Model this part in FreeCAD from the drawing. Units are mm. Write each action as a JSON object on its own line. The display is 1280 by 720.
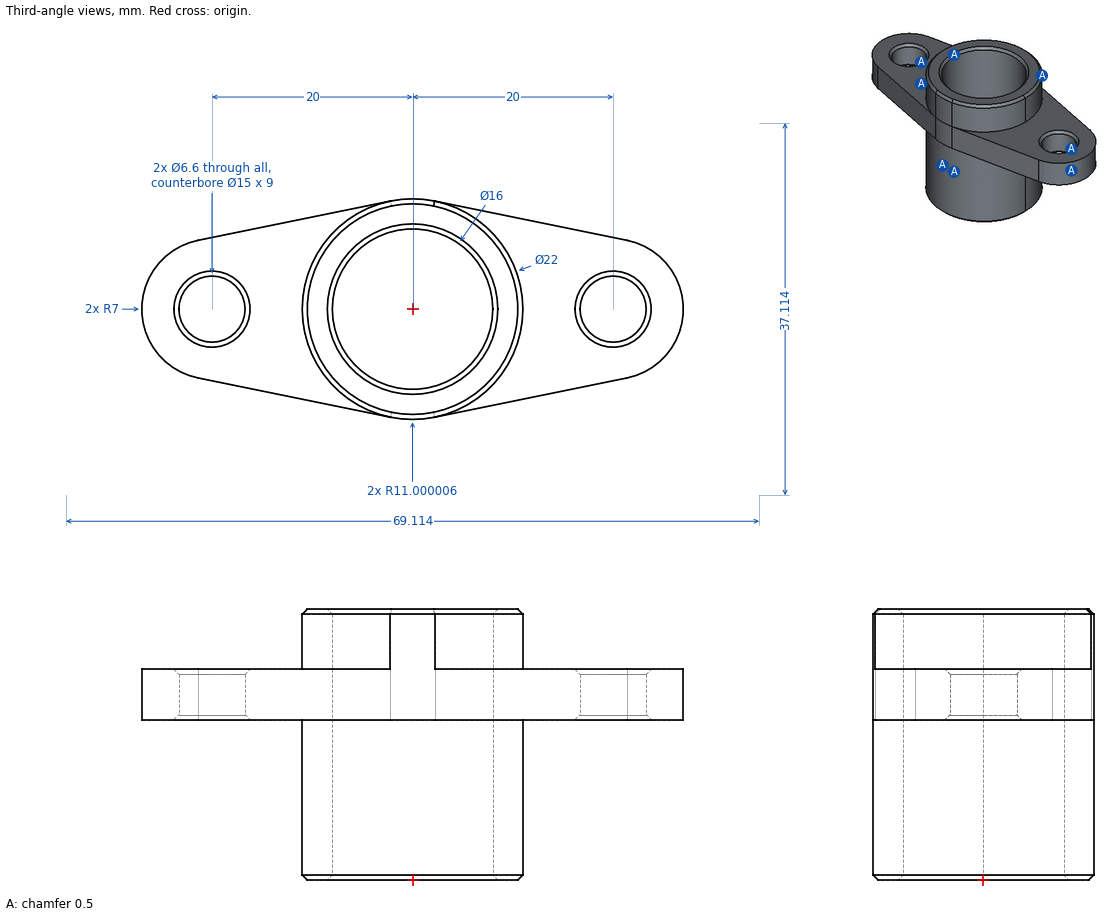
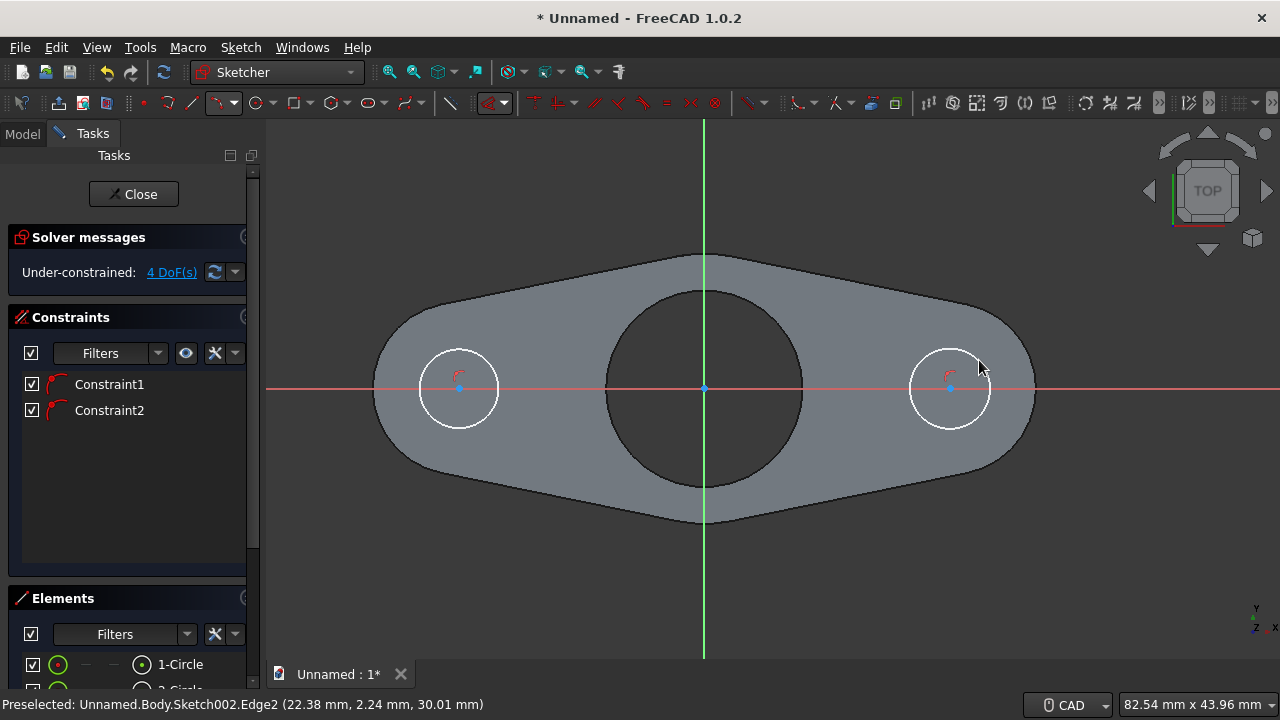
{"action": "left_click", "coordinate": [487, 361]}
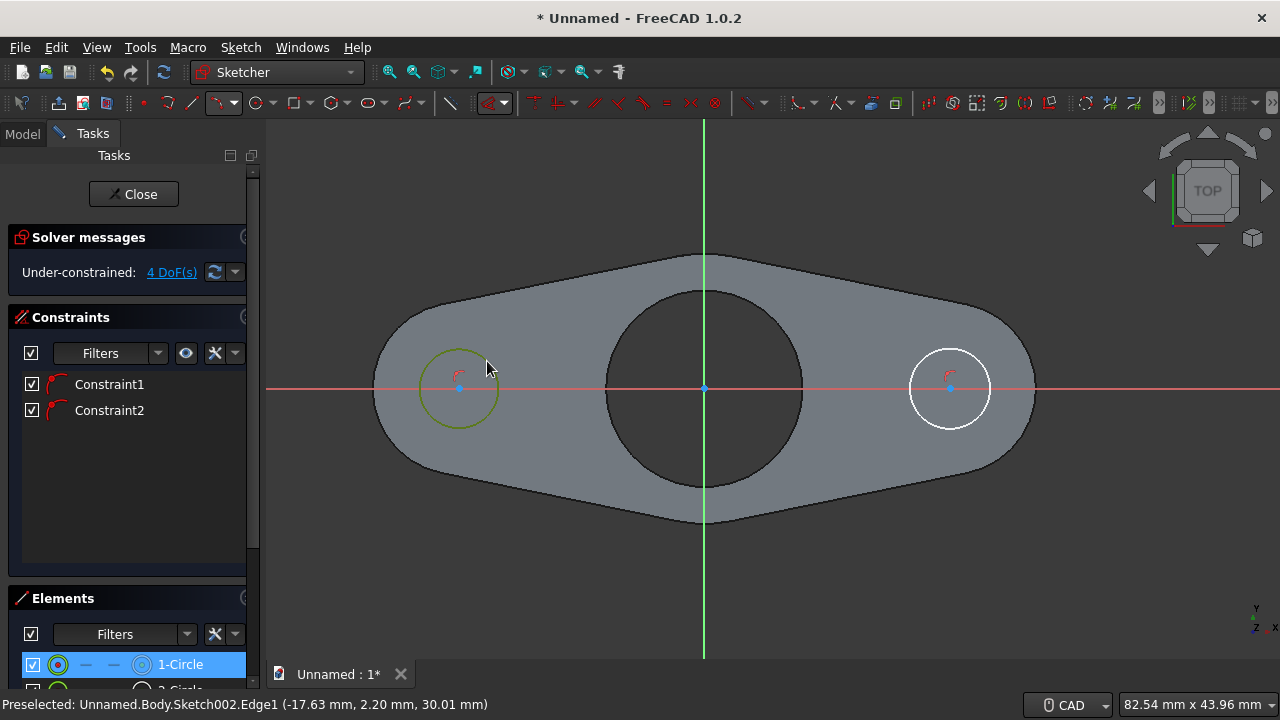
{"action": "left_click", "coordinate": [978, 360]}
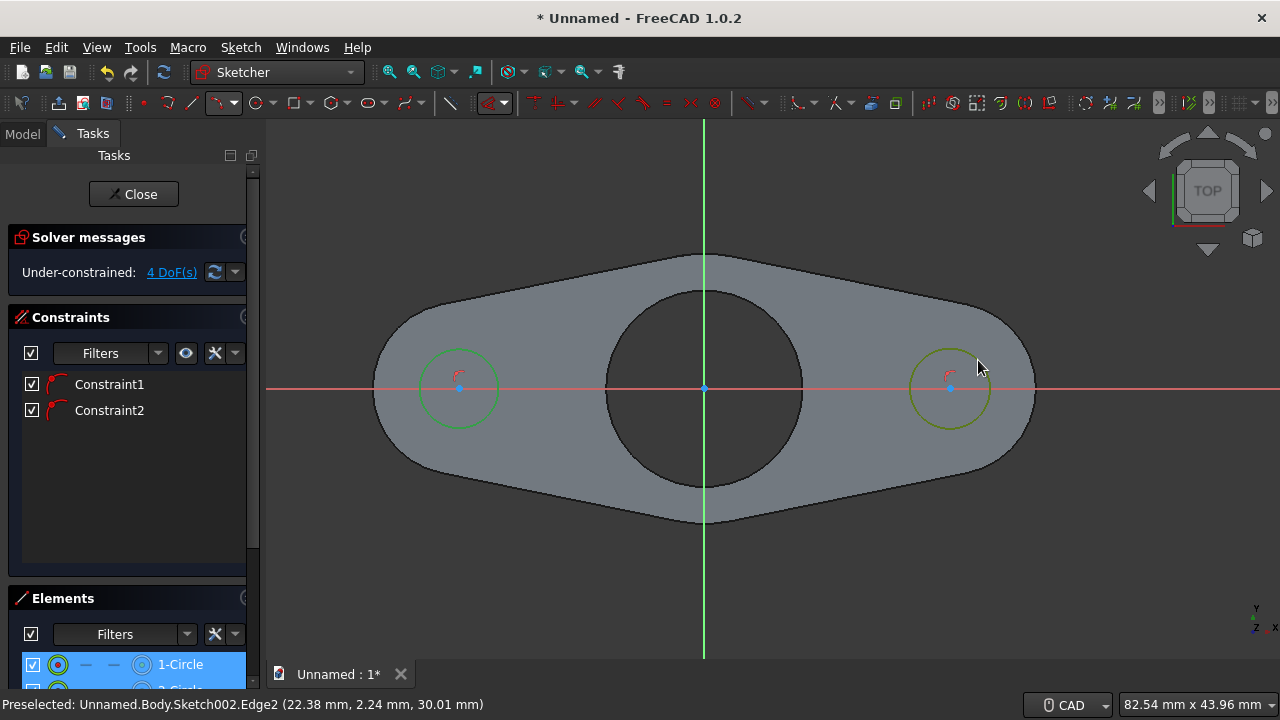
{"action": "left_click", "coordinate": [668, 104]}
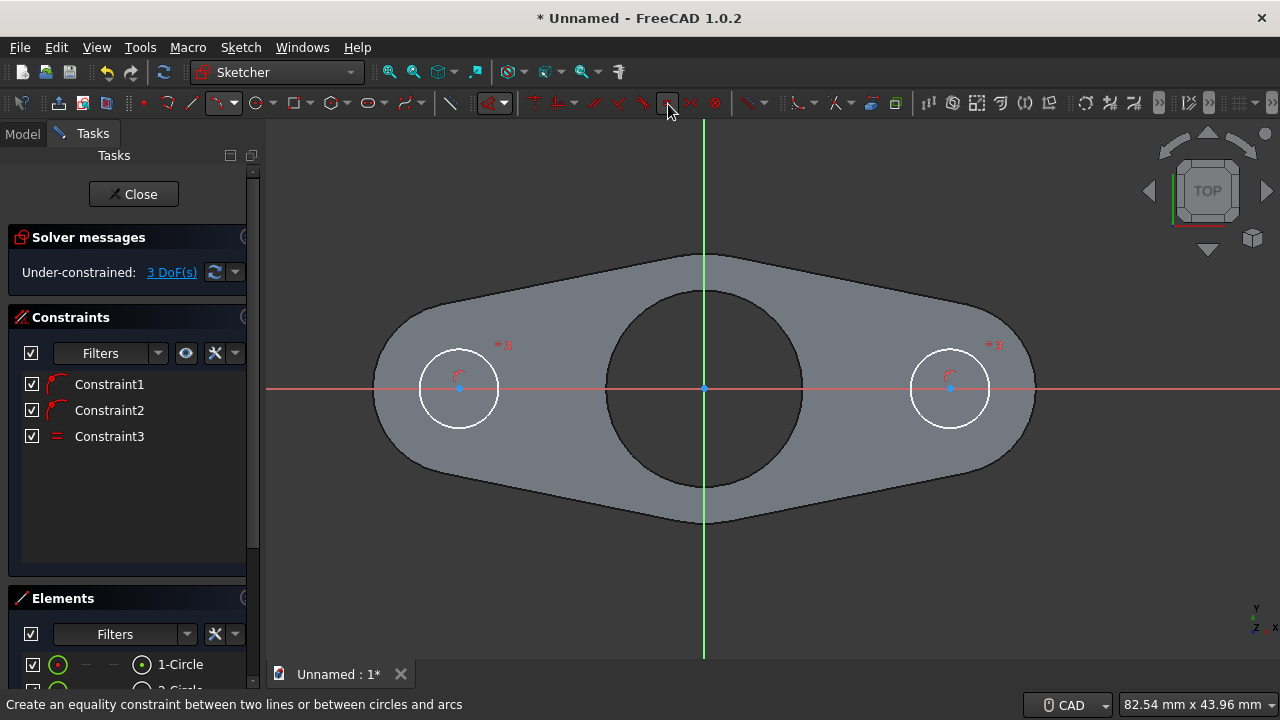
{"action": "left_click", "coordinate": [487, 361]}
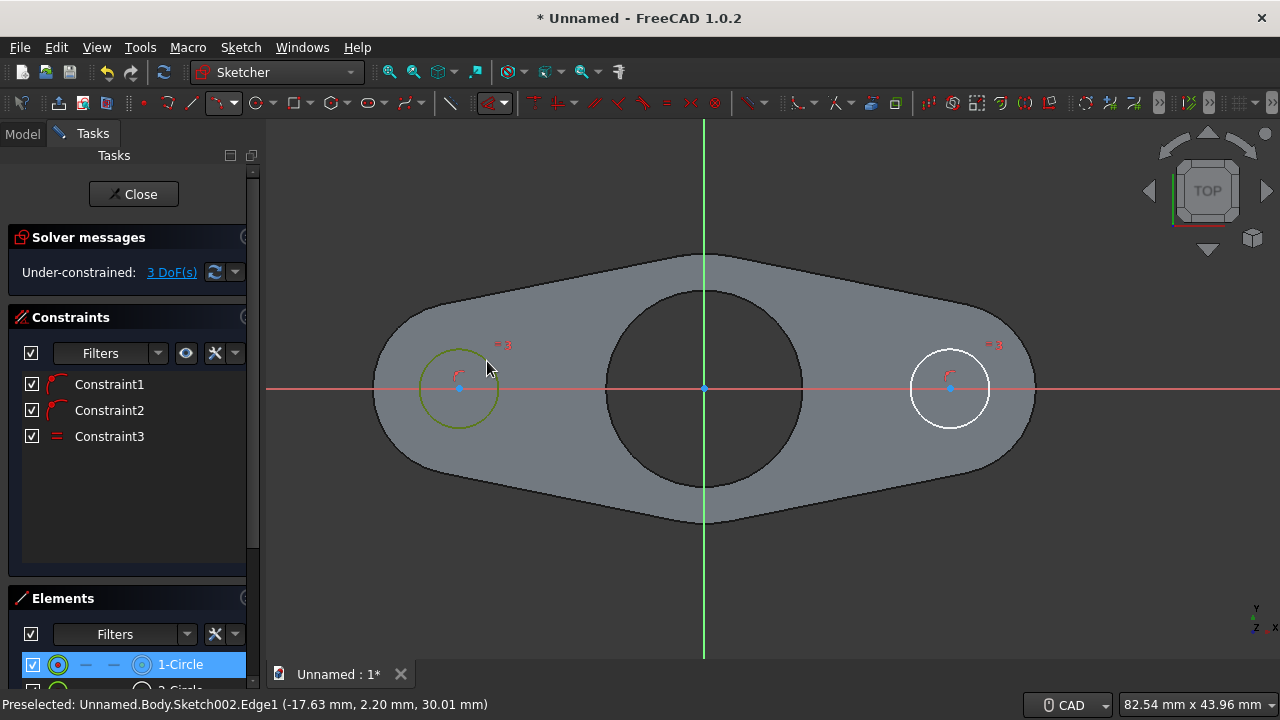
{"action": "key", "text": "k o"}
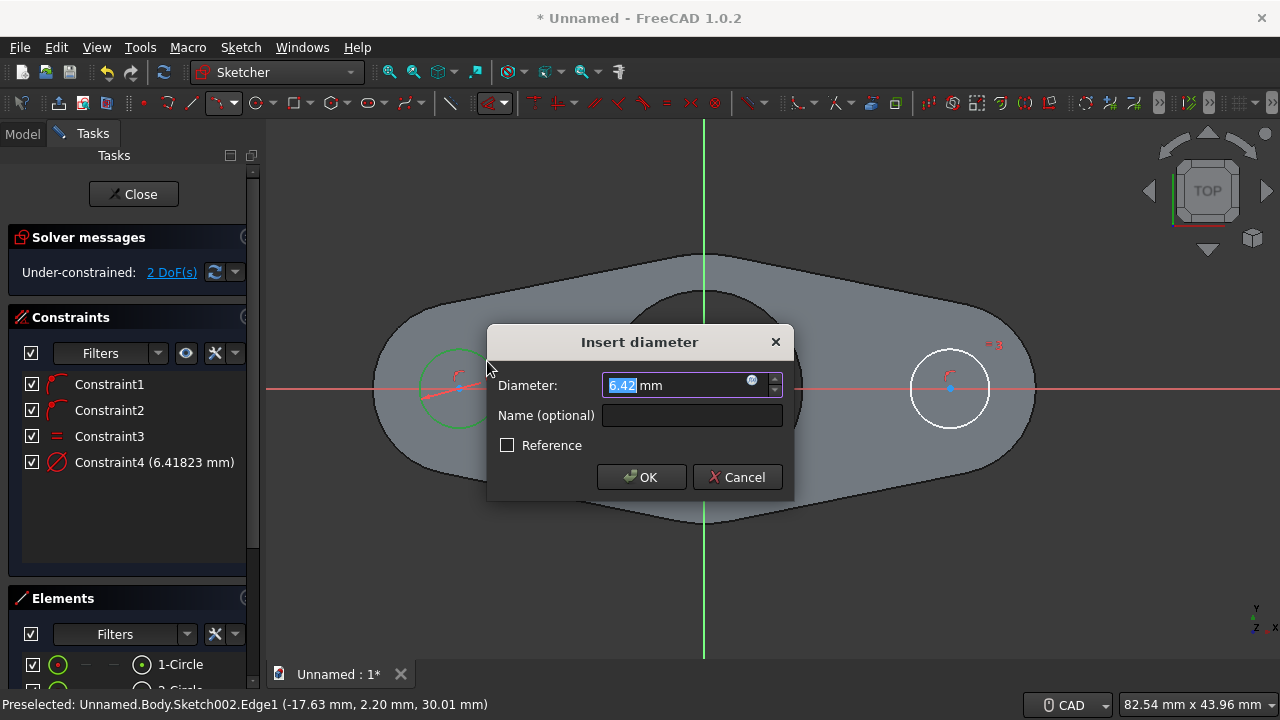
{"action": "type", "text": "6.6"}
{"action": "key", "text": "Return"}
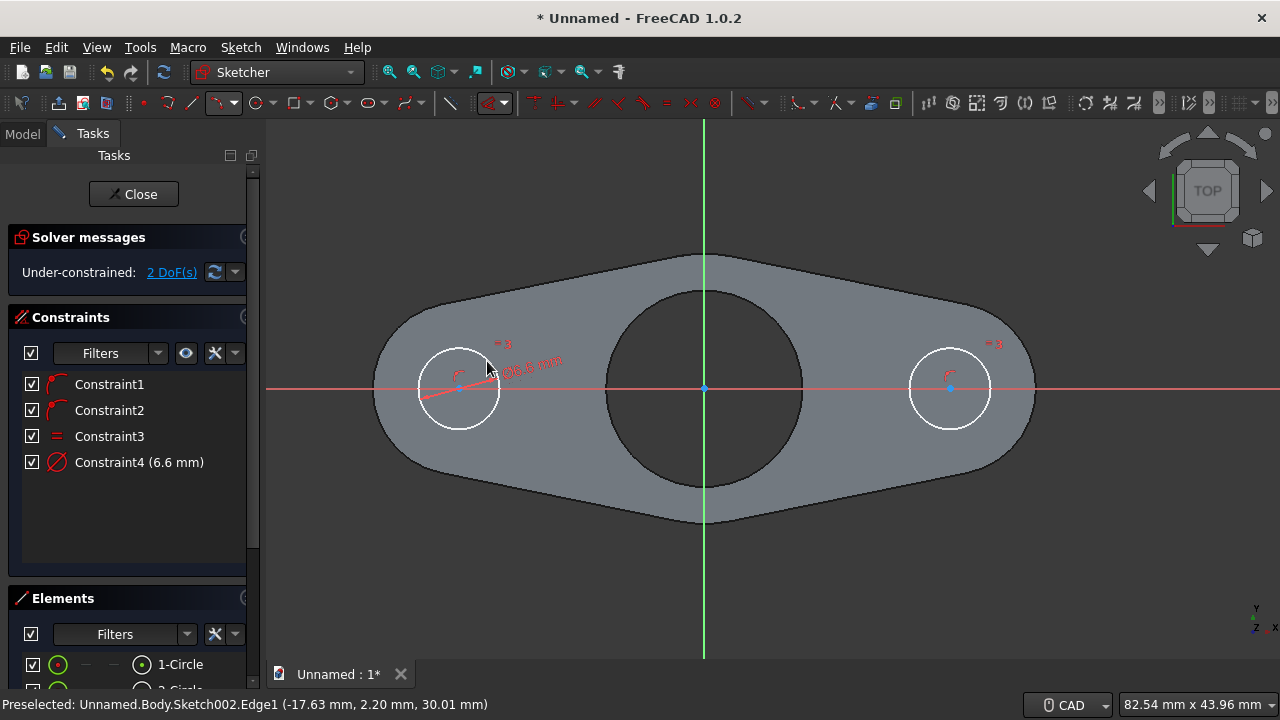
{"action": "left_click", "coordinate": [459, 389]}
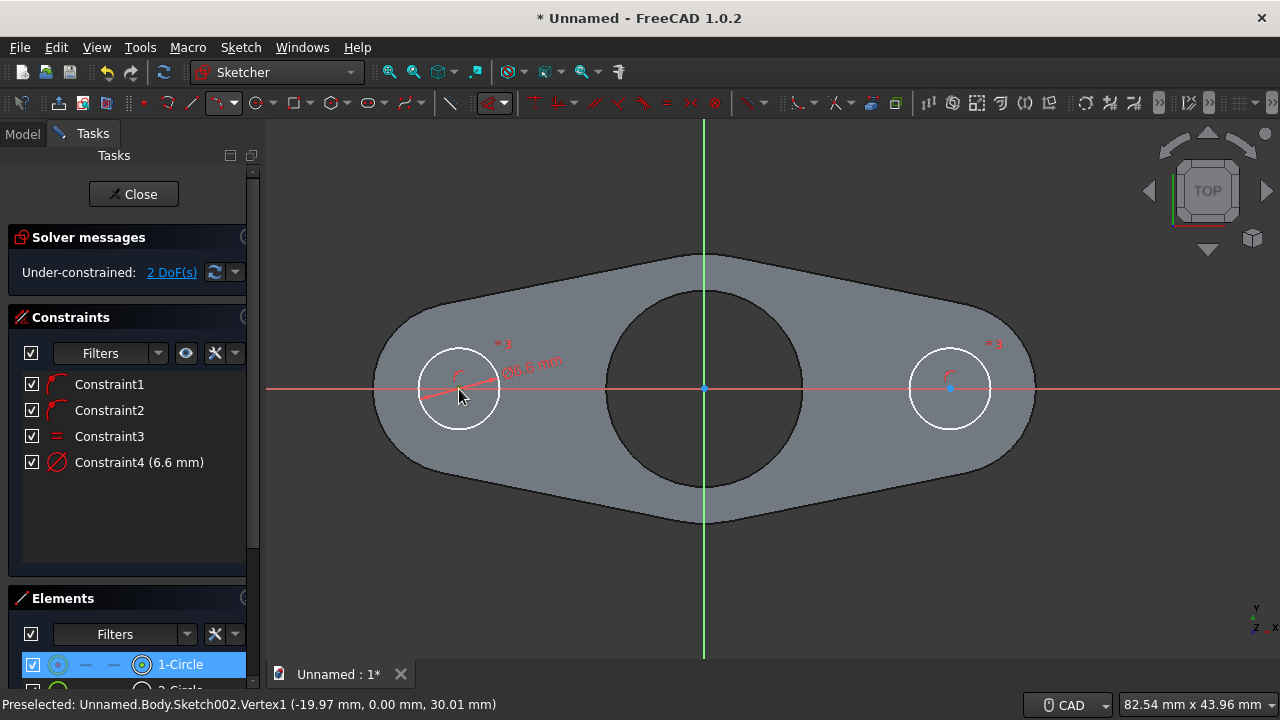
{"action": "key", "text": "l"}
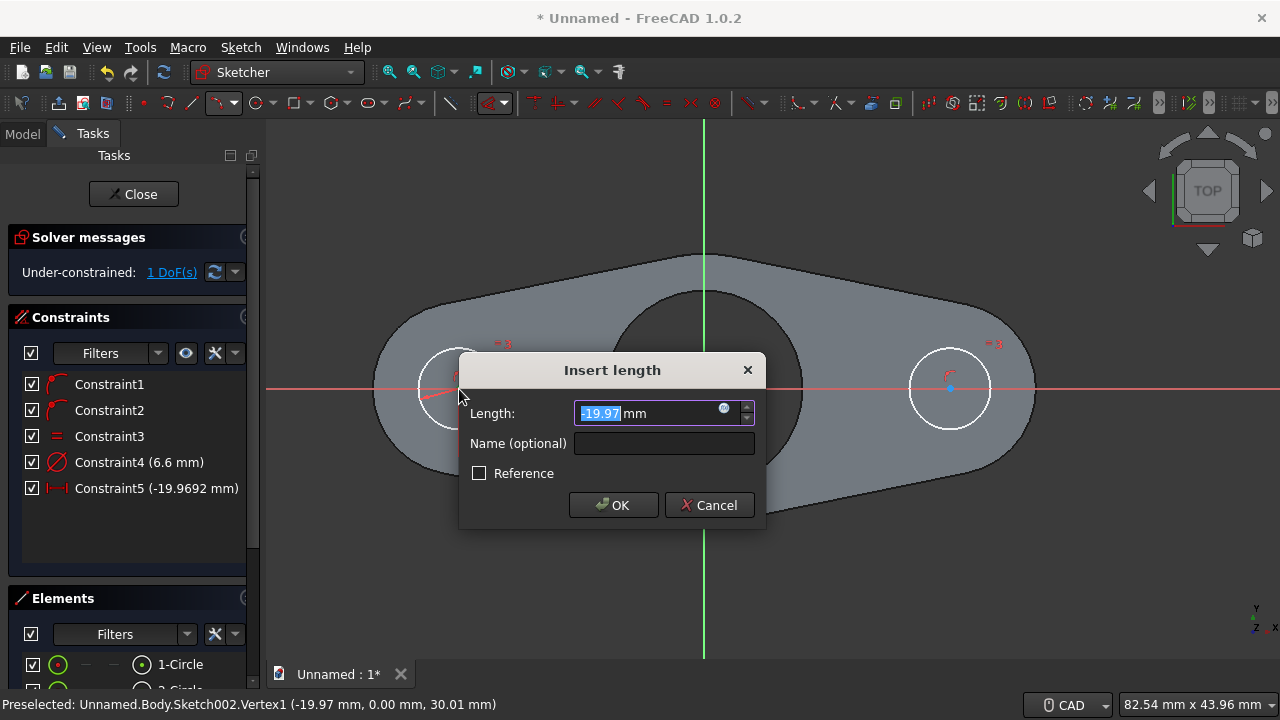
{"action": "type", "text": "-20"}
{"action": "key", "text": "Return"}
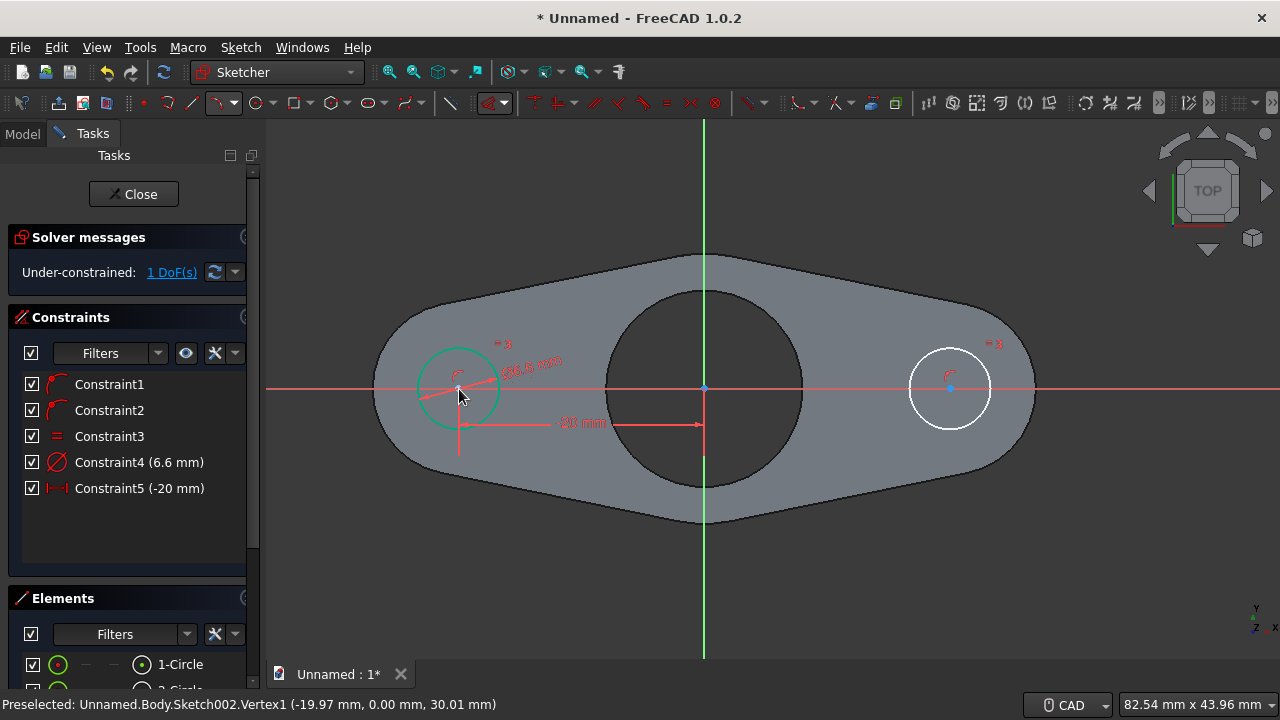
{"action": "left_click", "coordinate": [950, 389]}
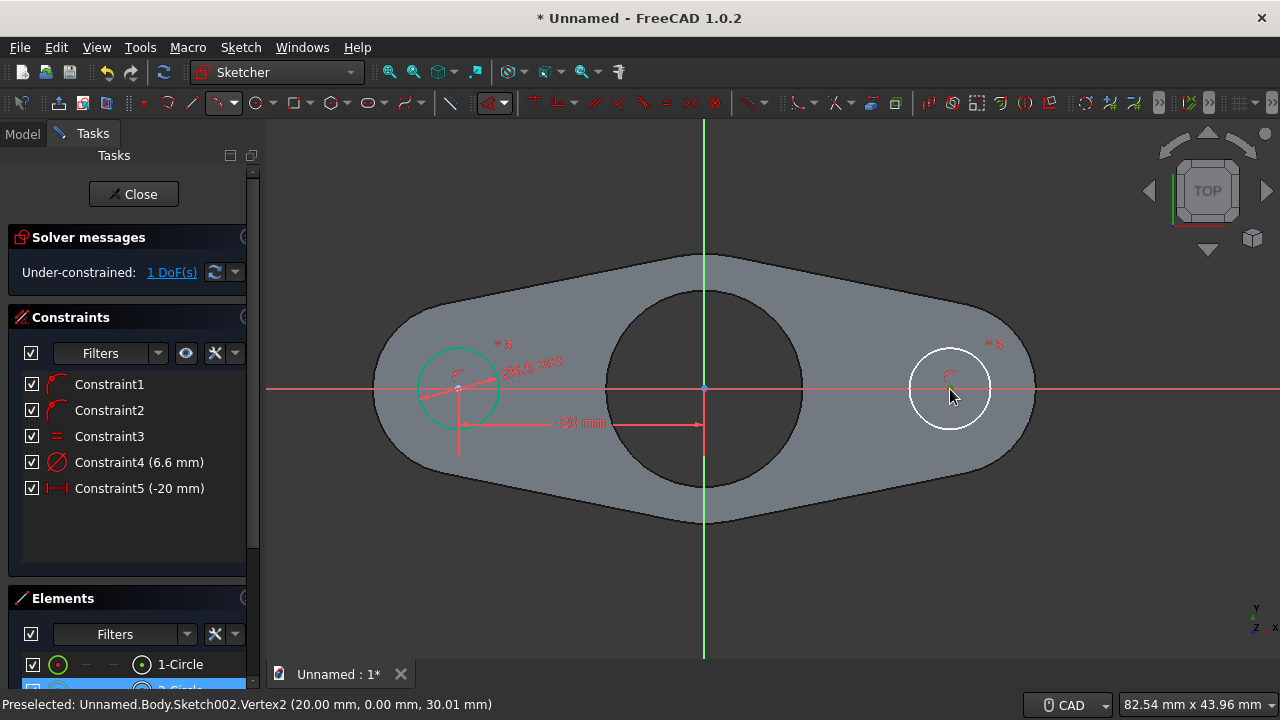
{"action": "key", "text": "l"}